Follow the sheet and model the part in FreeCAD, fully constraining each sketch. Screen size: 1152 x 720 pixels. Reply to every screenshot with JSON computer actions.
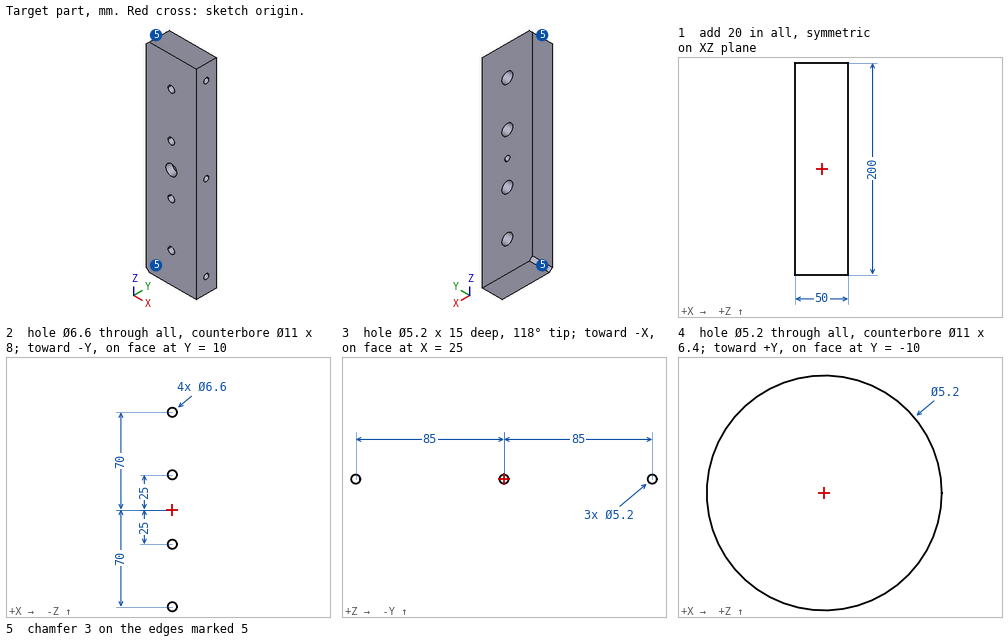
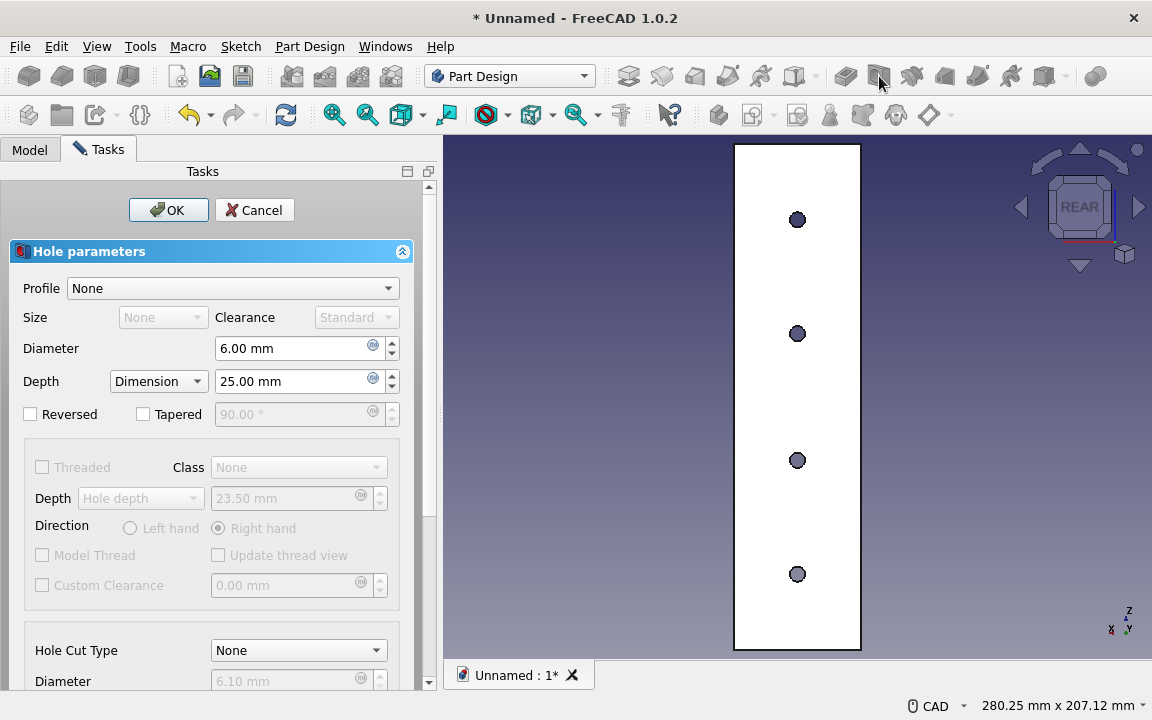
{"action": "triple_click", "coordinate": [300, 348]}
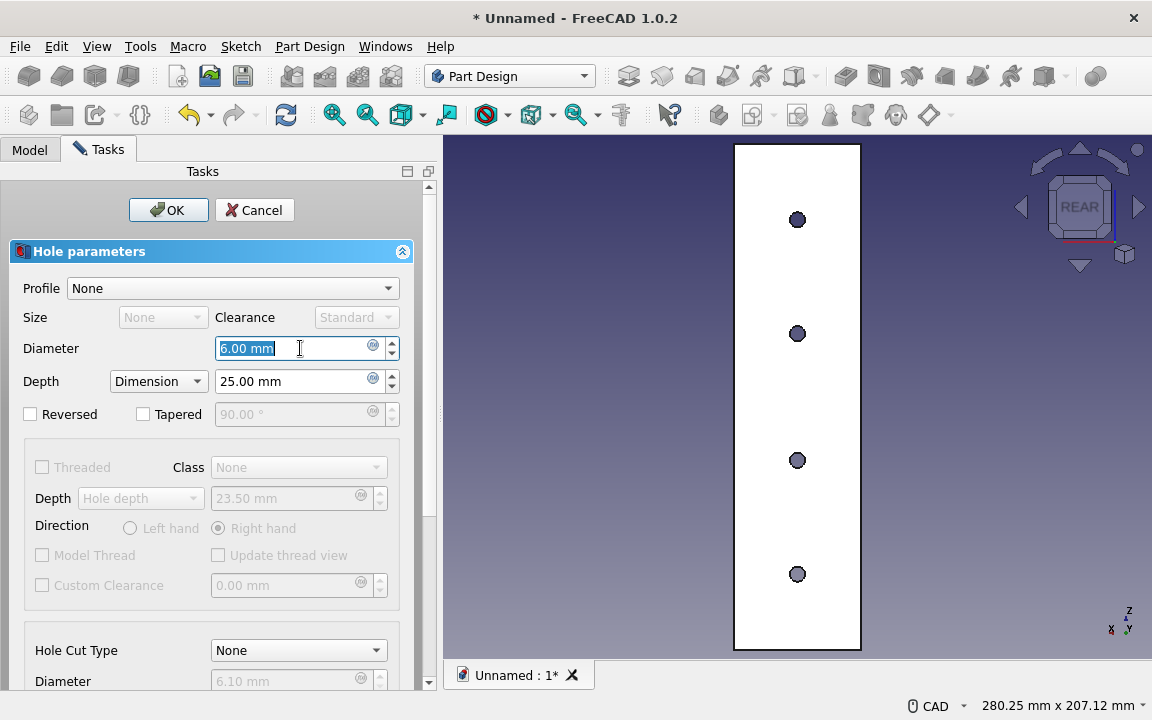
{"action": "type", "text": "6.6"}
{"action": "key", "text": "Tab"}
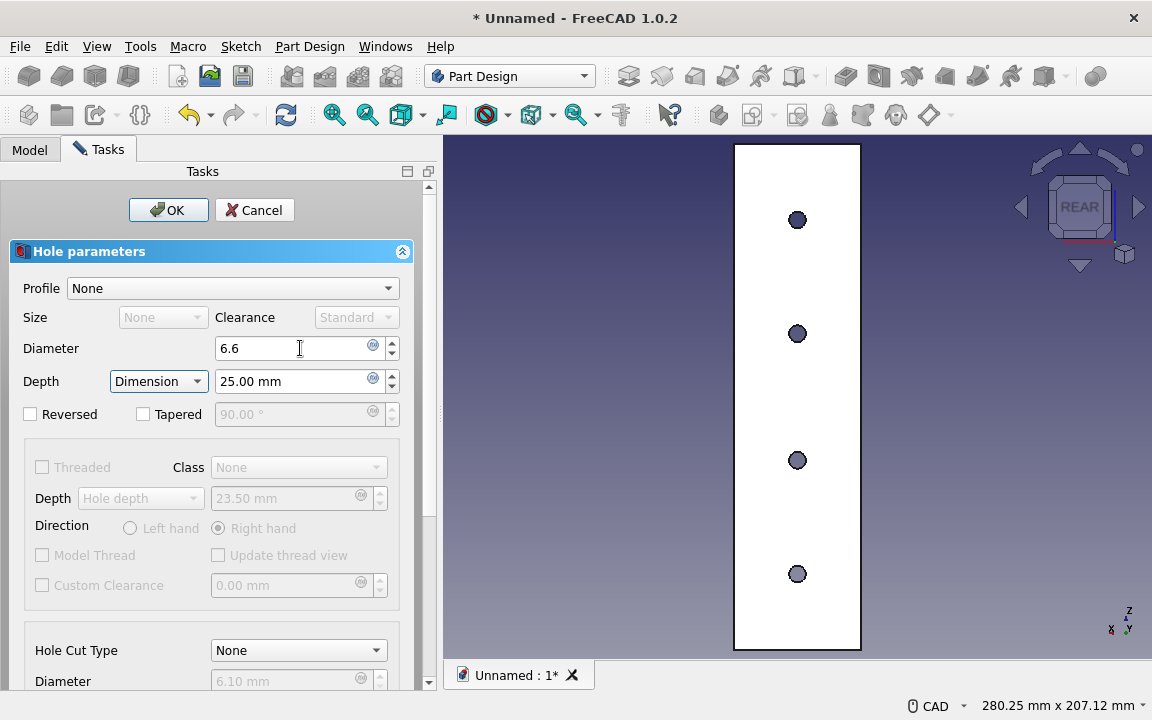
{"action": "left_click", "coordinate": [160, 382]}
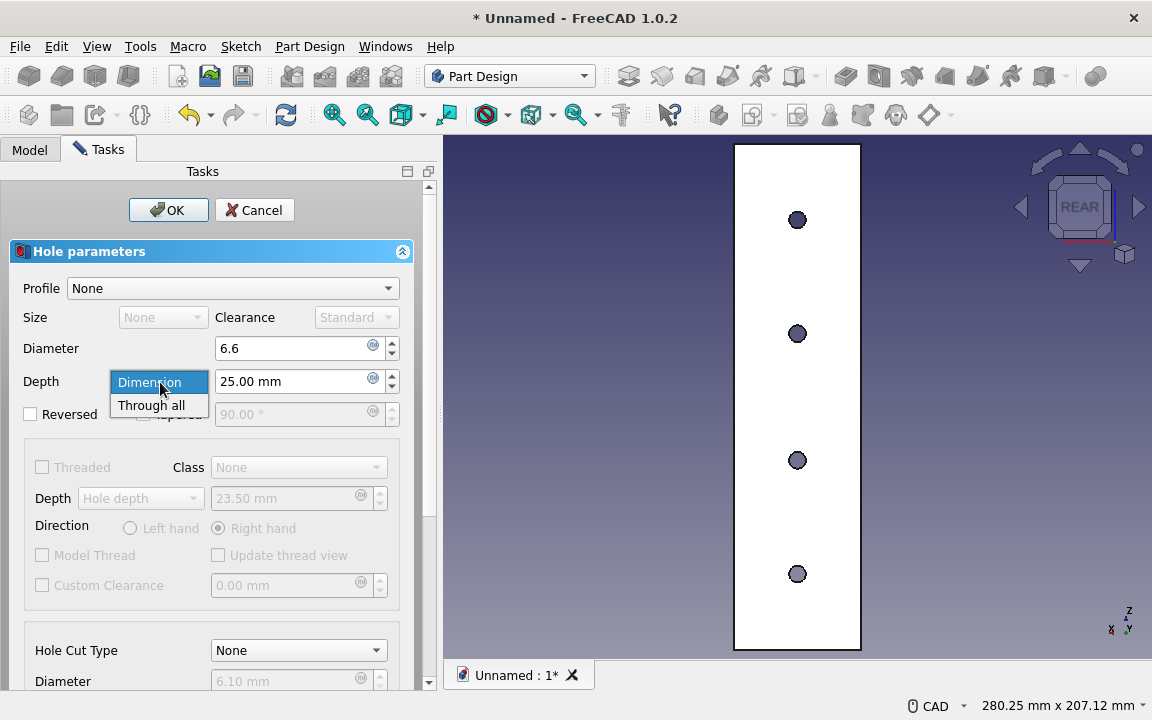
{"action": "left_click", "coordinate": [158, 406]}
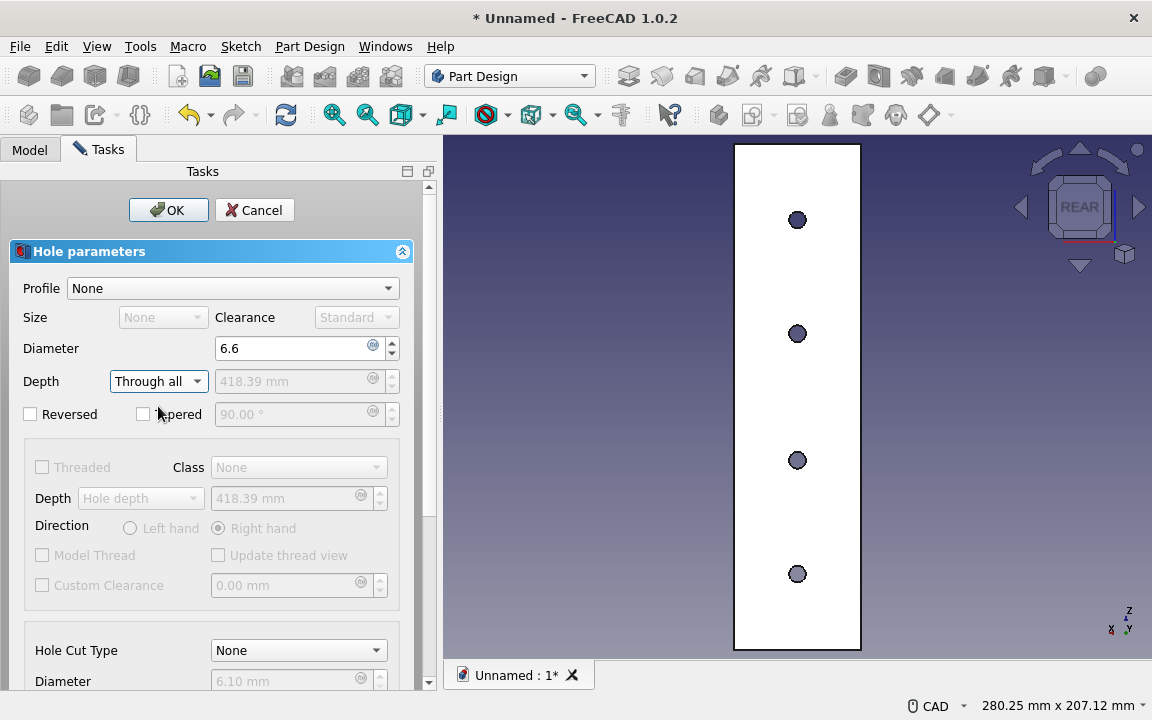
{"action": "left_click", "coordinate": [300, 650]}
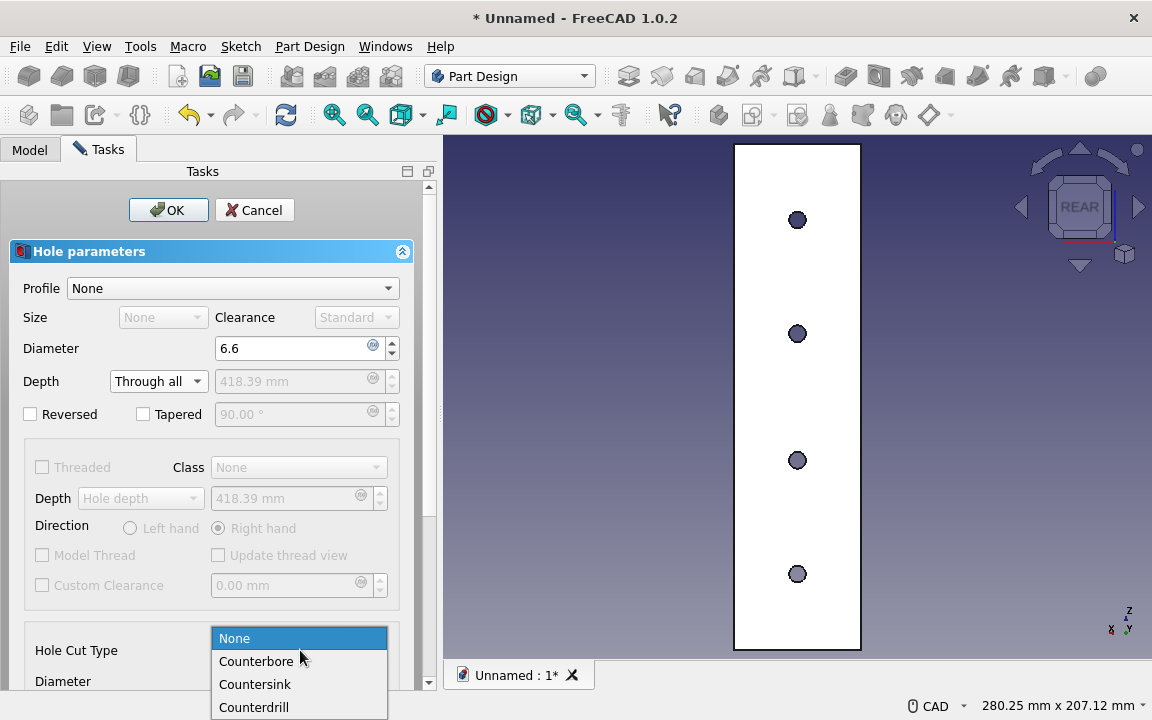
{"action": "left_click", "coordinate": [298, 662]}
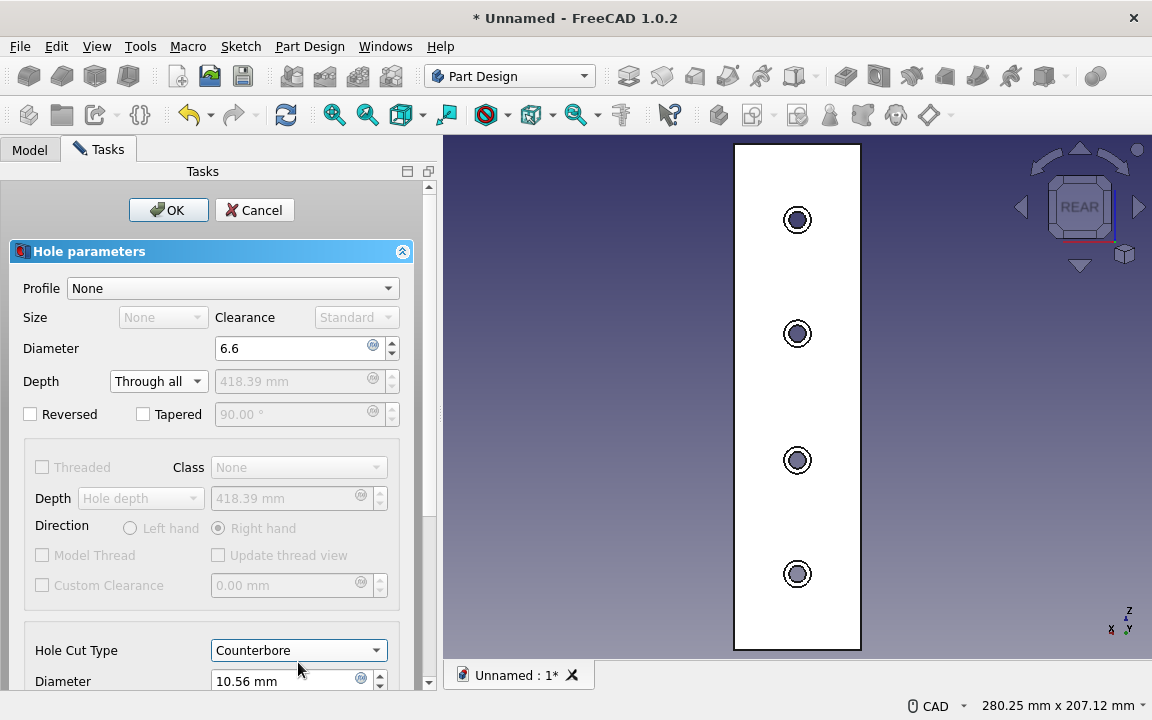
{"action": "scroll", "coordinate": [429, 436], "scroll_direction": "down", "scroll_amount": 2}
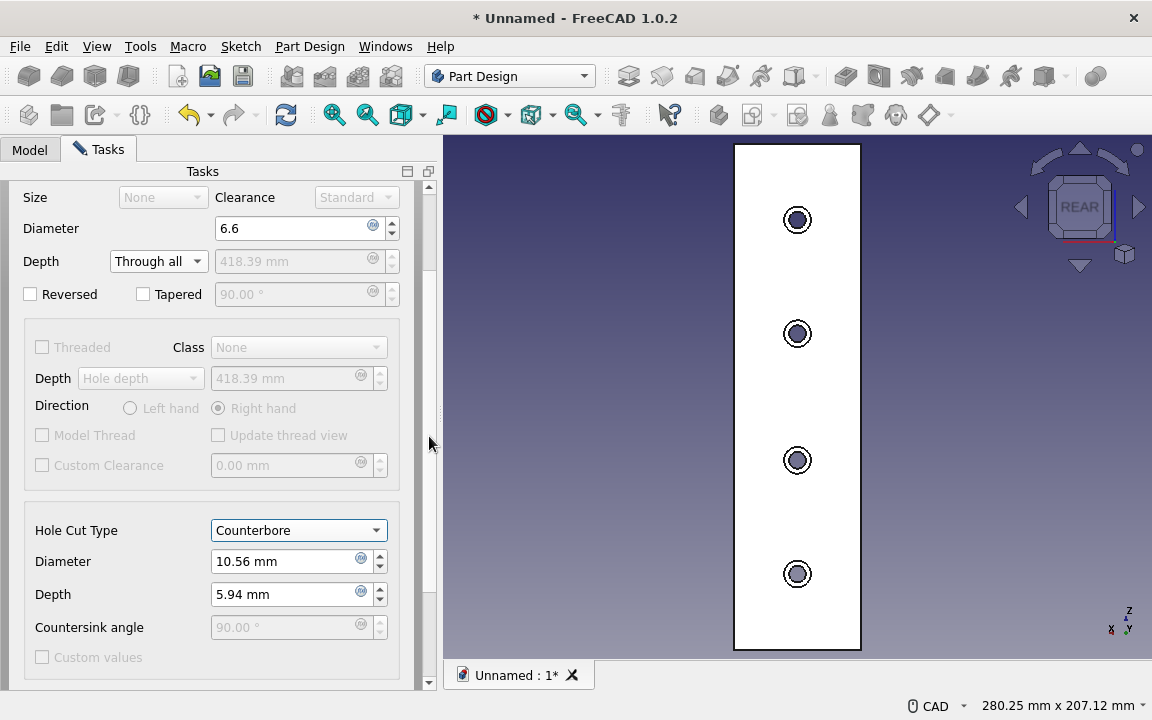
{"action": "triple_click", "coordinate": [292, 562]}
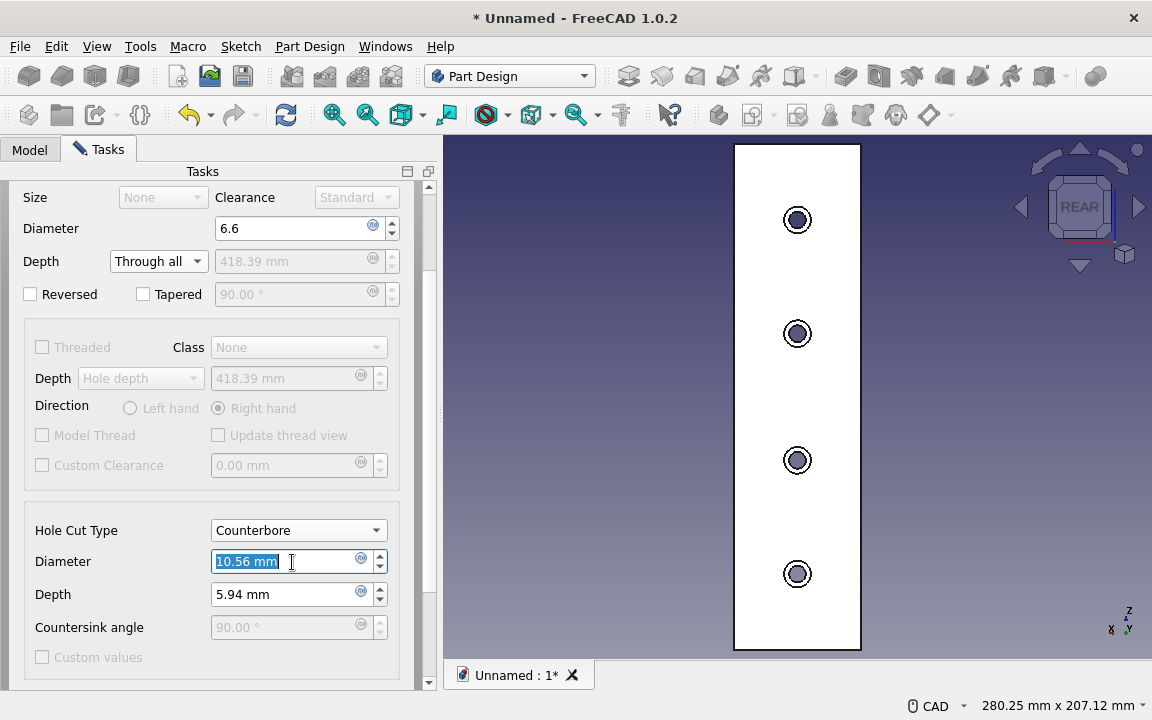
{"action": "type", "text": "11"}
{"action": "key", "text": "Tab"}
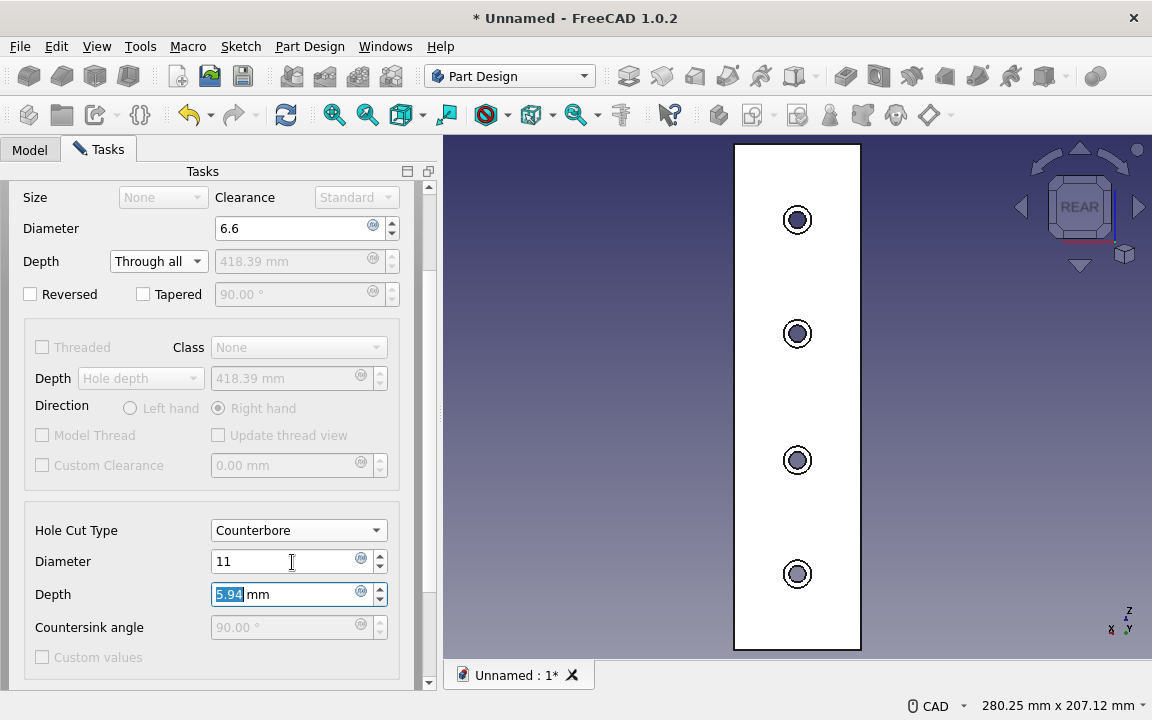
{"action": "type", "text": "8"}
{"action": "key", "text": "Tab"}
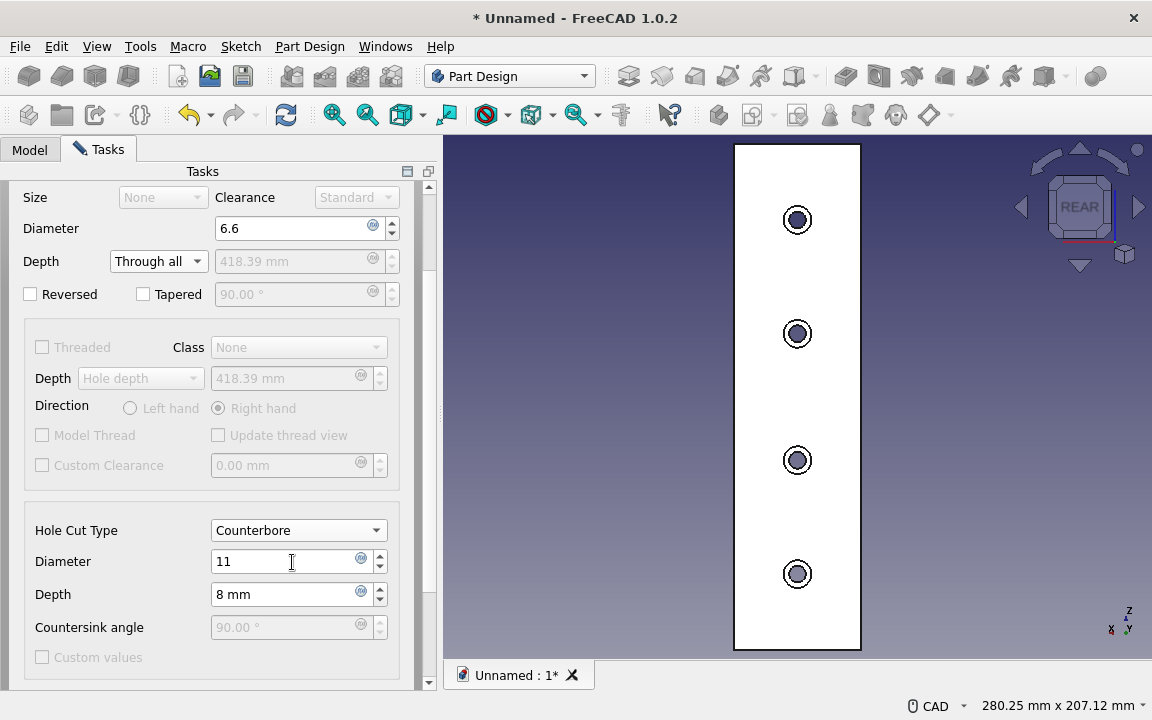
{"action": "scroll", "coordinate": [429, 436], "scroll_direction": "up", "scroll_amount": 3}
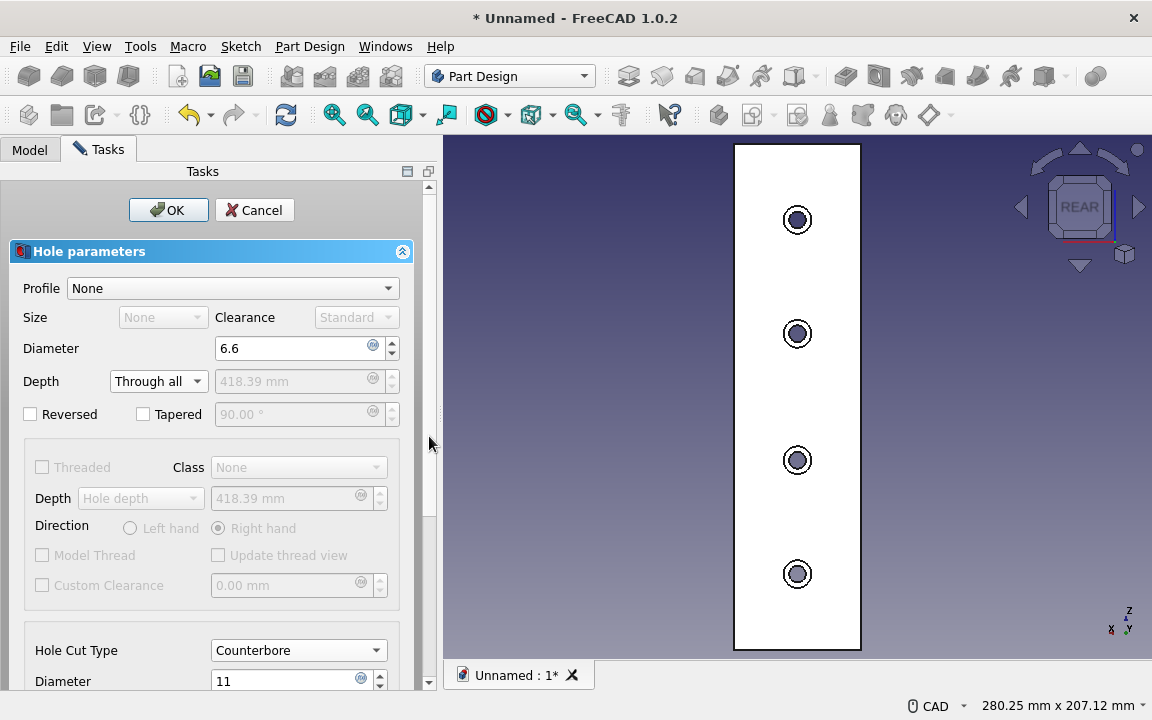
{"action": "left_click", "coordinate": [169, 210]}